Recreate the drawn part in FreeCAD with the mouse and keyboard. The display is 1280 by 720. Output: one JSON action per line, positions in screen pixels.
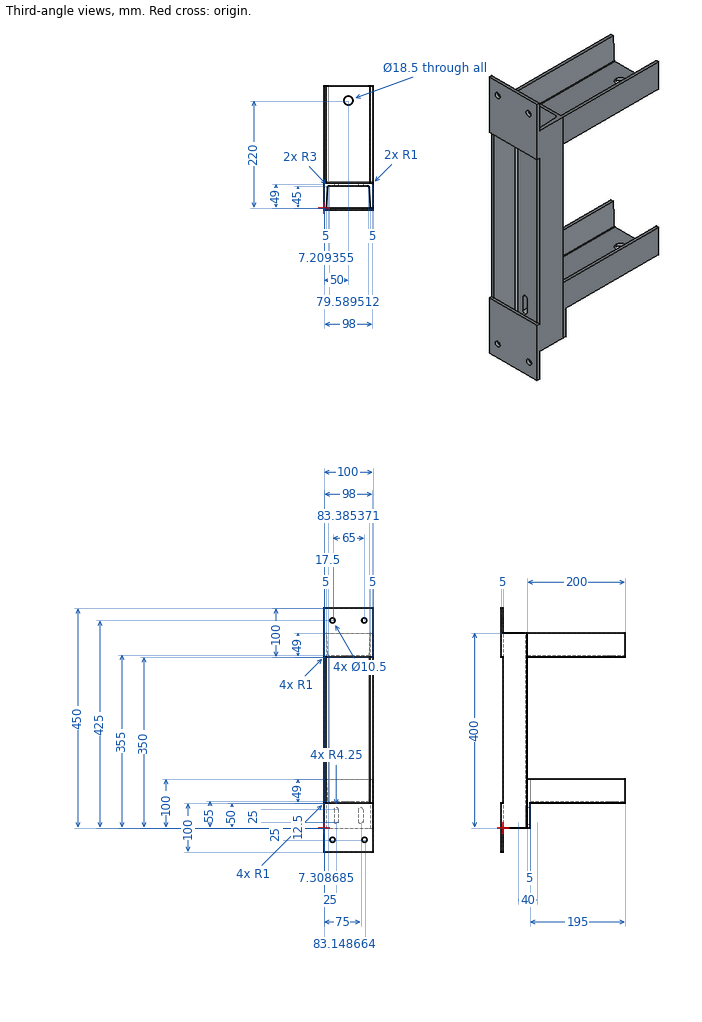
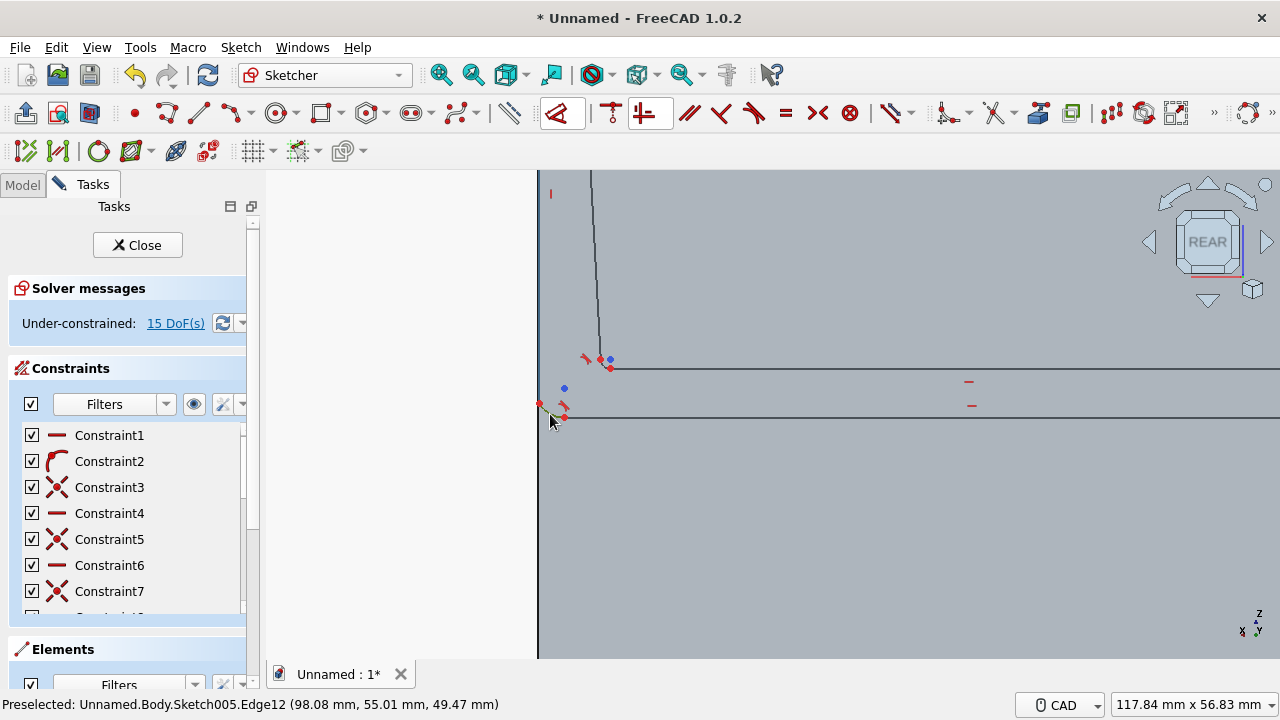
{"action": "left_click", "coordinate": [754, 114]}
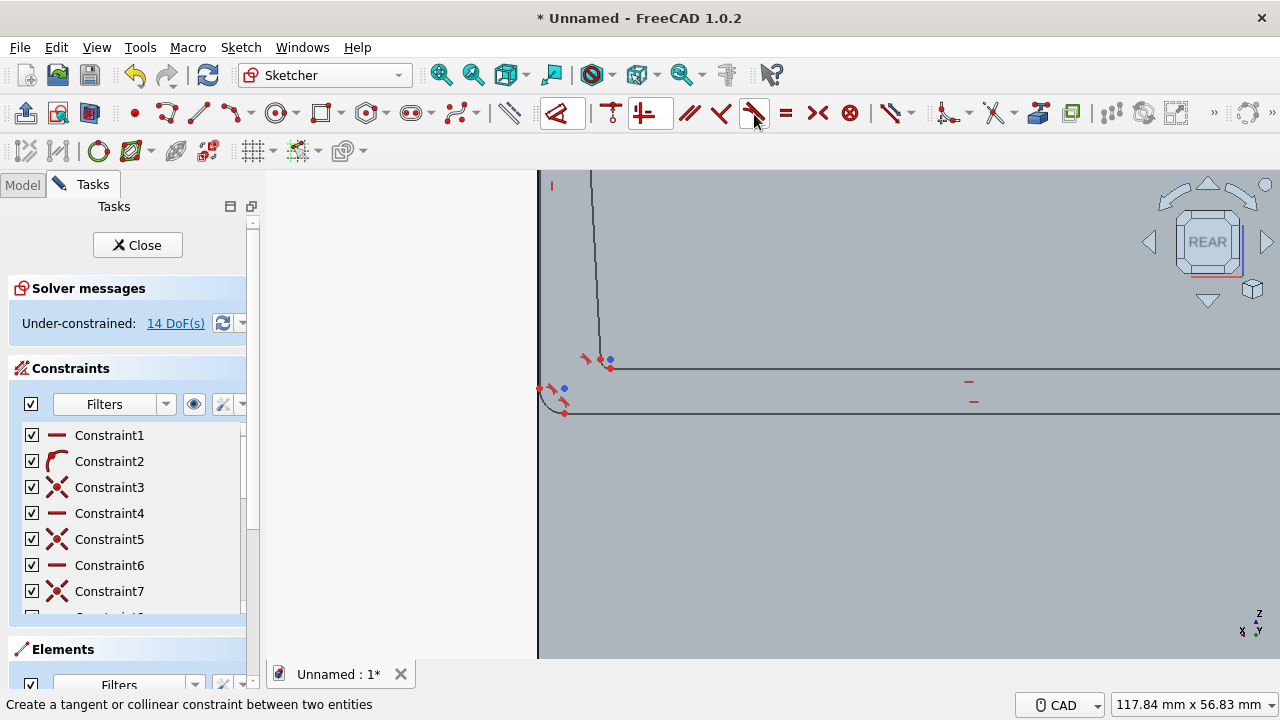
{"action": "scroll", "coordinate": [551, 416], "scroll_direction": "down", "scroll_amount": 5}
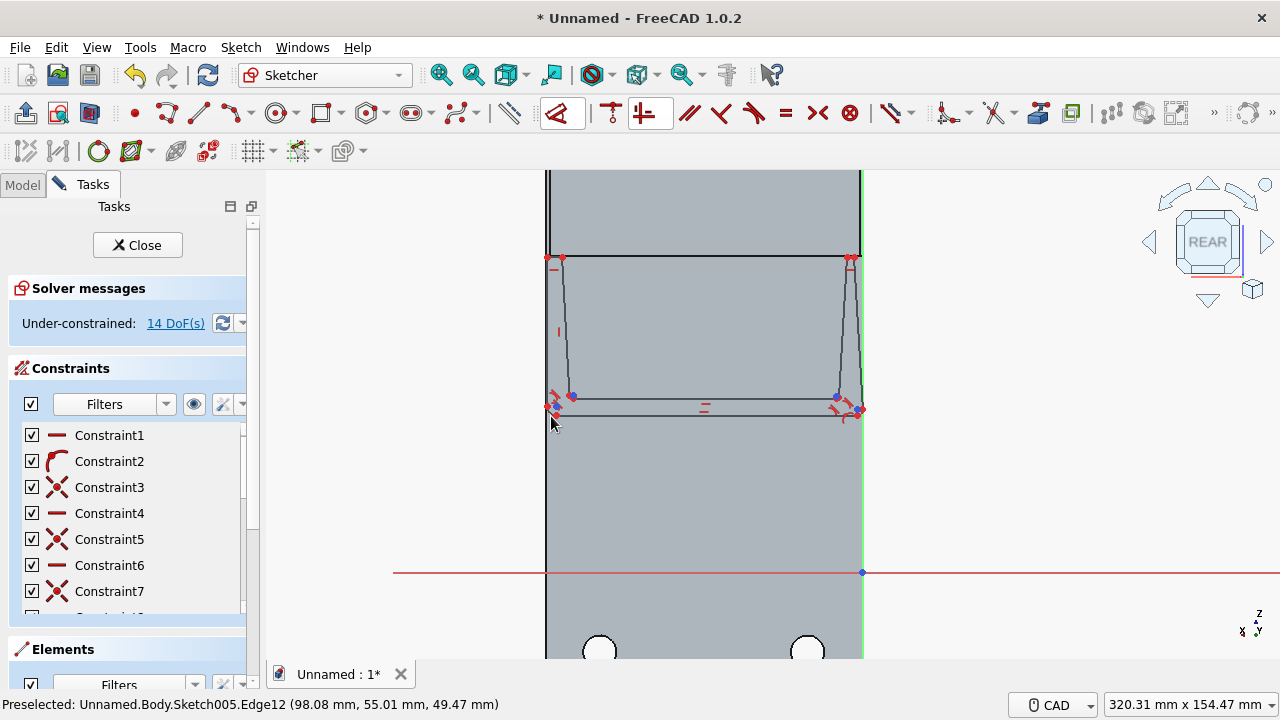
{"action": "scroll", "coordinate": [857, 303], "scroll_direction": "up", "scroll_amount": 4}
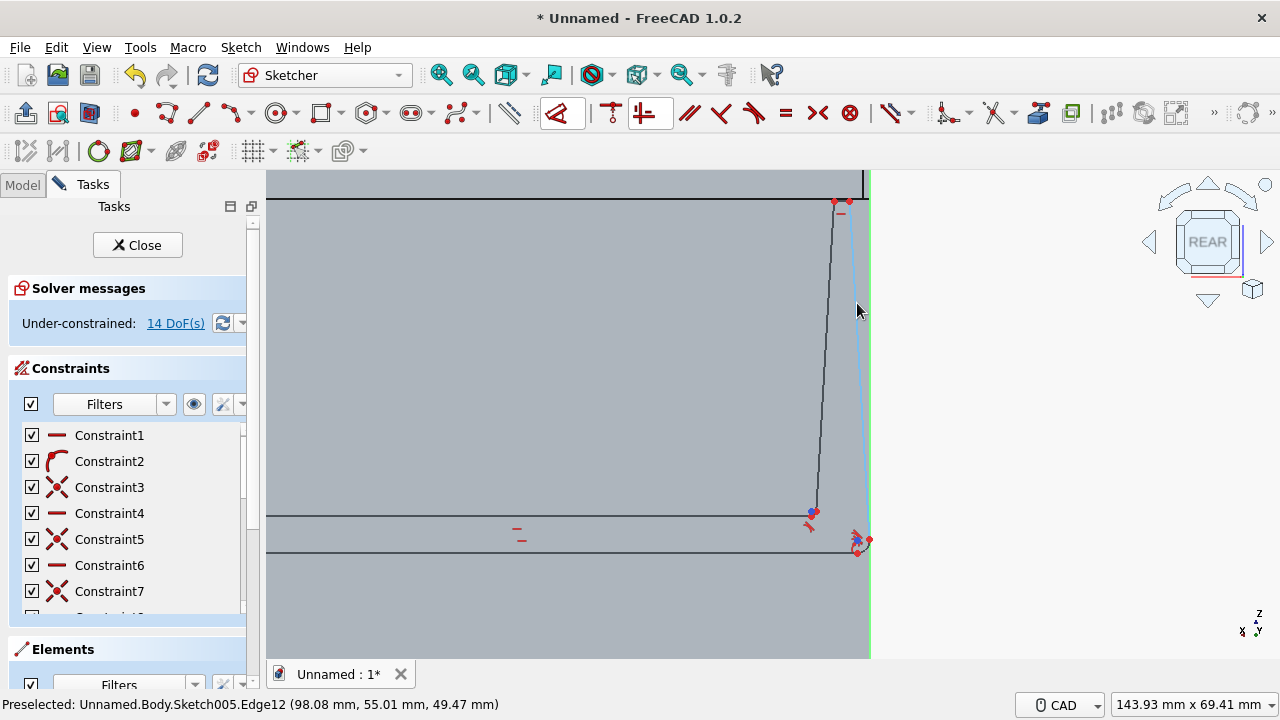
{"action": "left_click", "coordinate": [856, 303]}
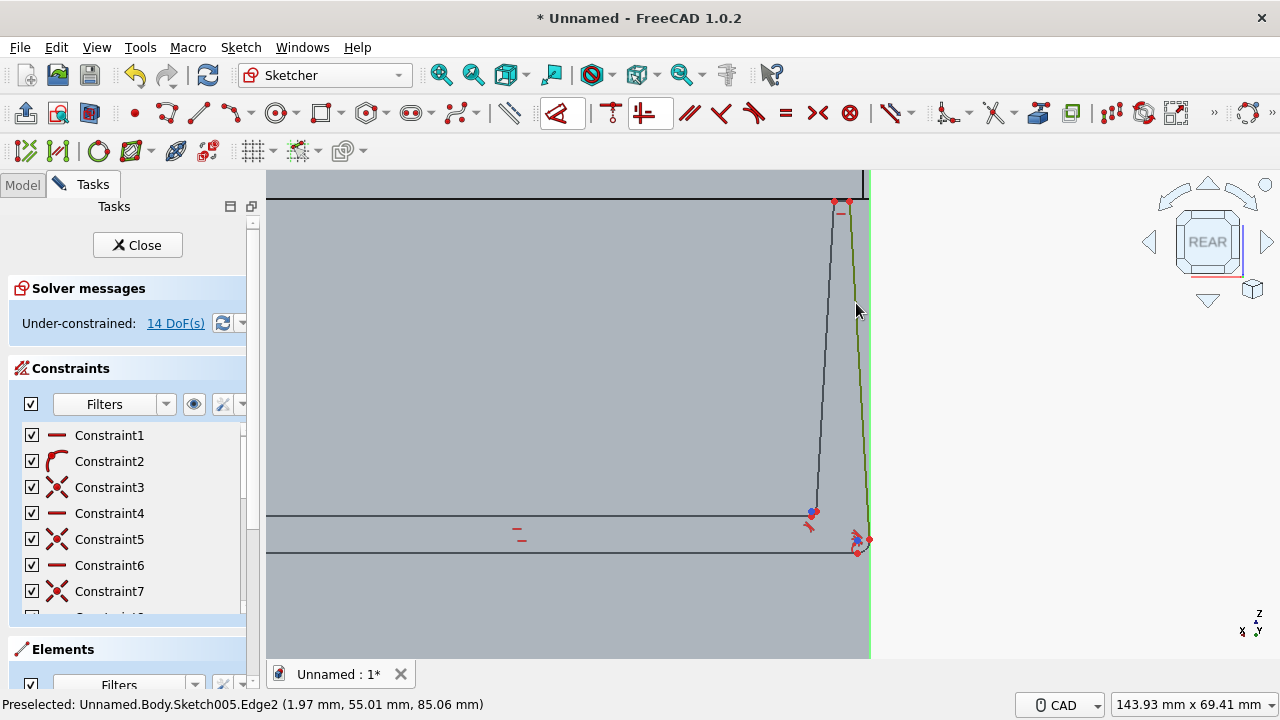
{"action": "left_click", "coordinate": [668, 114]}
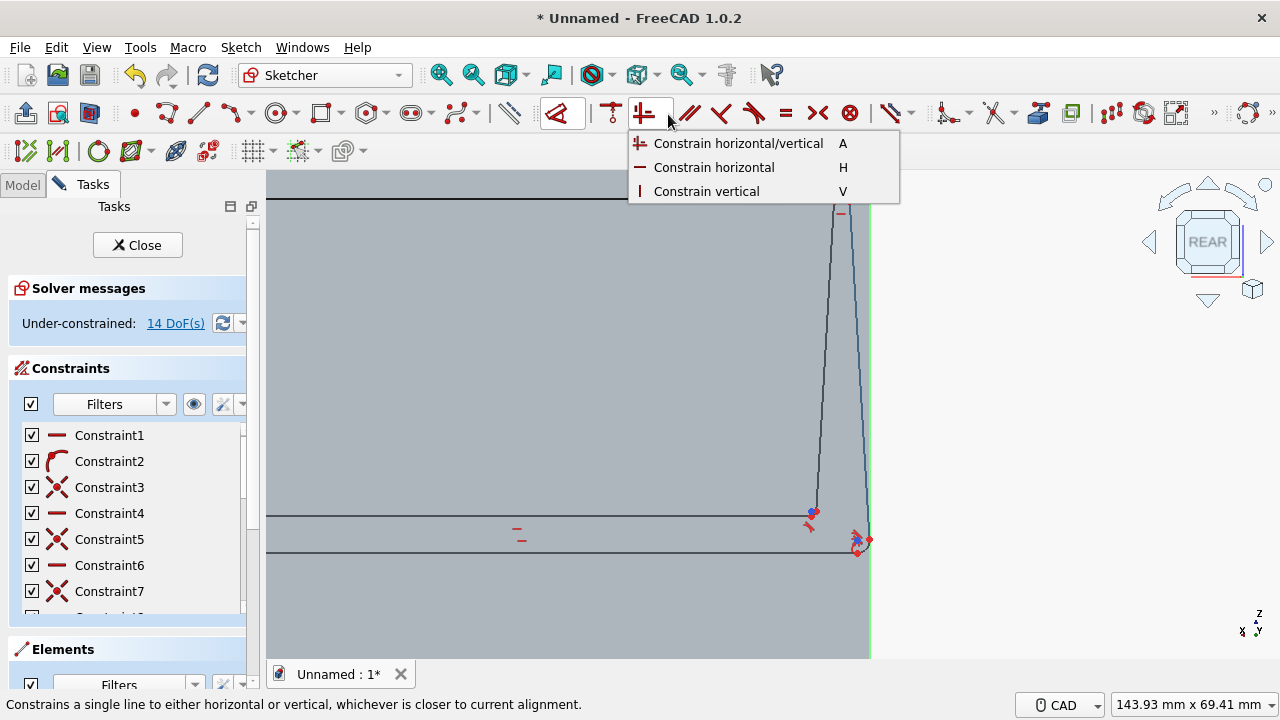
{"action": "left_click", "coordinate": [764, 191]}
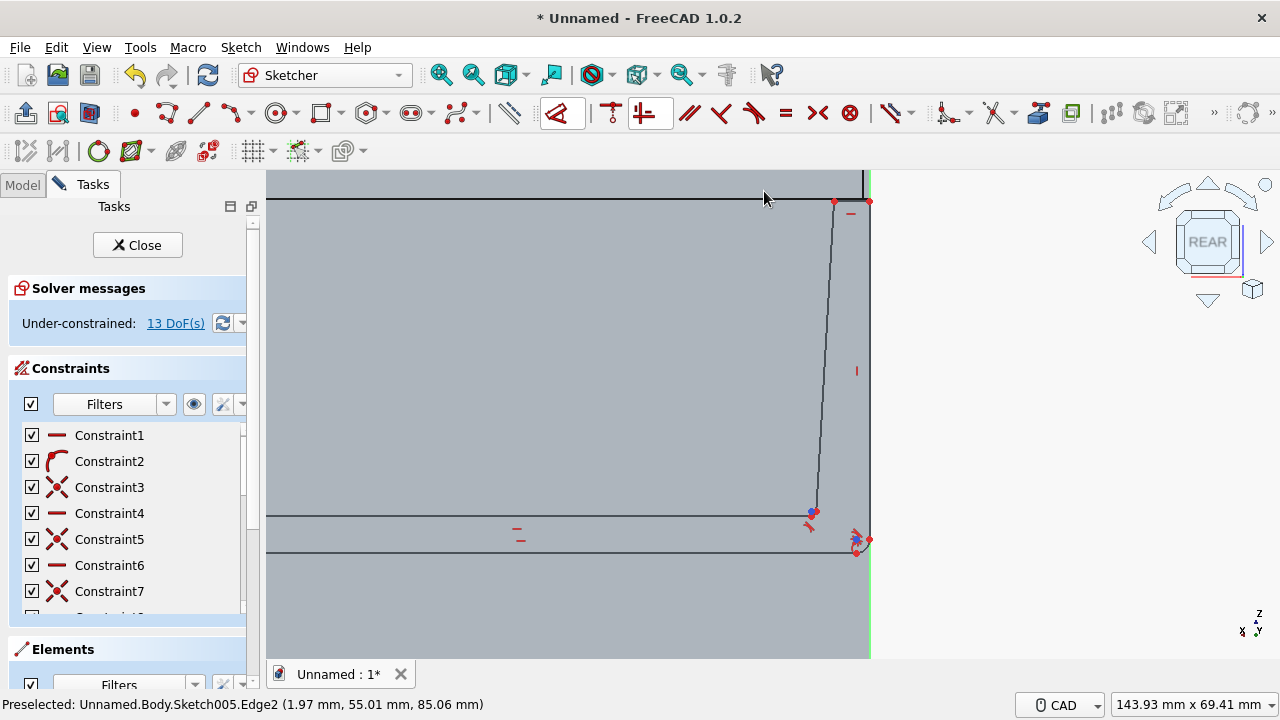
{"action": "scroll", "coordinate": [866, 549], "scroll_direction": "up", "scroll_amount": 2}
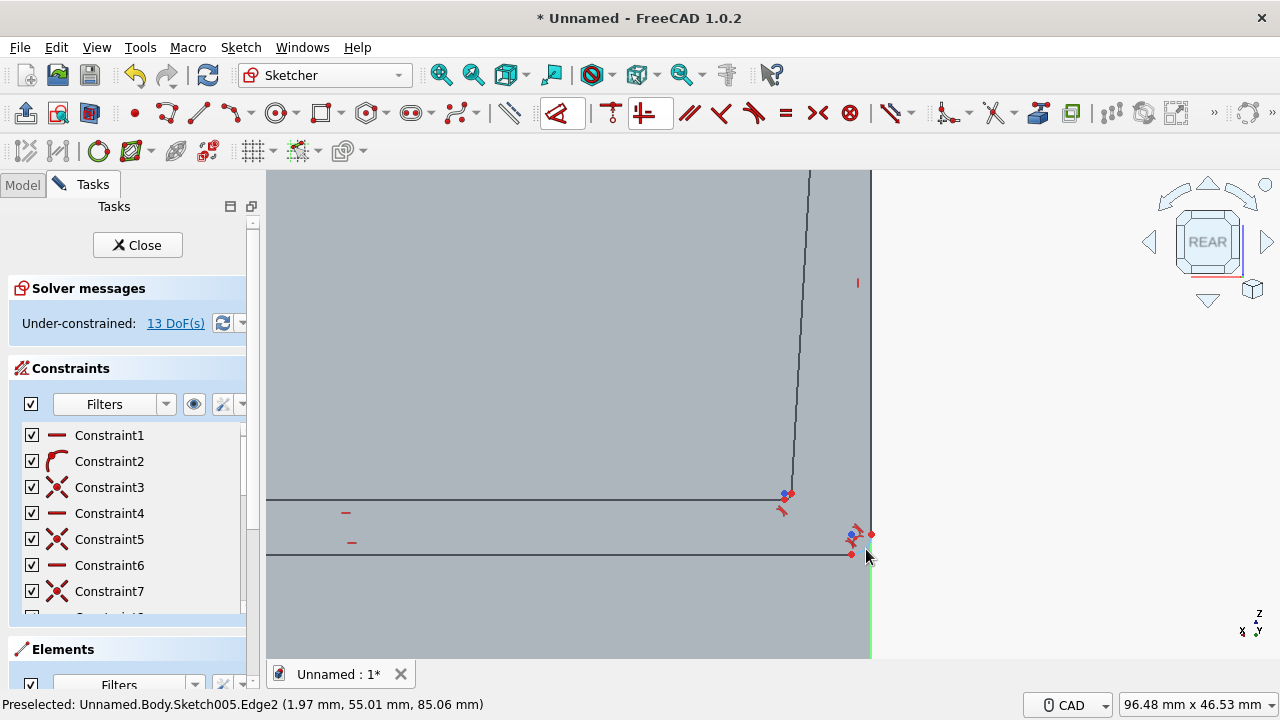
{"action": "left_click", "coordinate": [865, 549]}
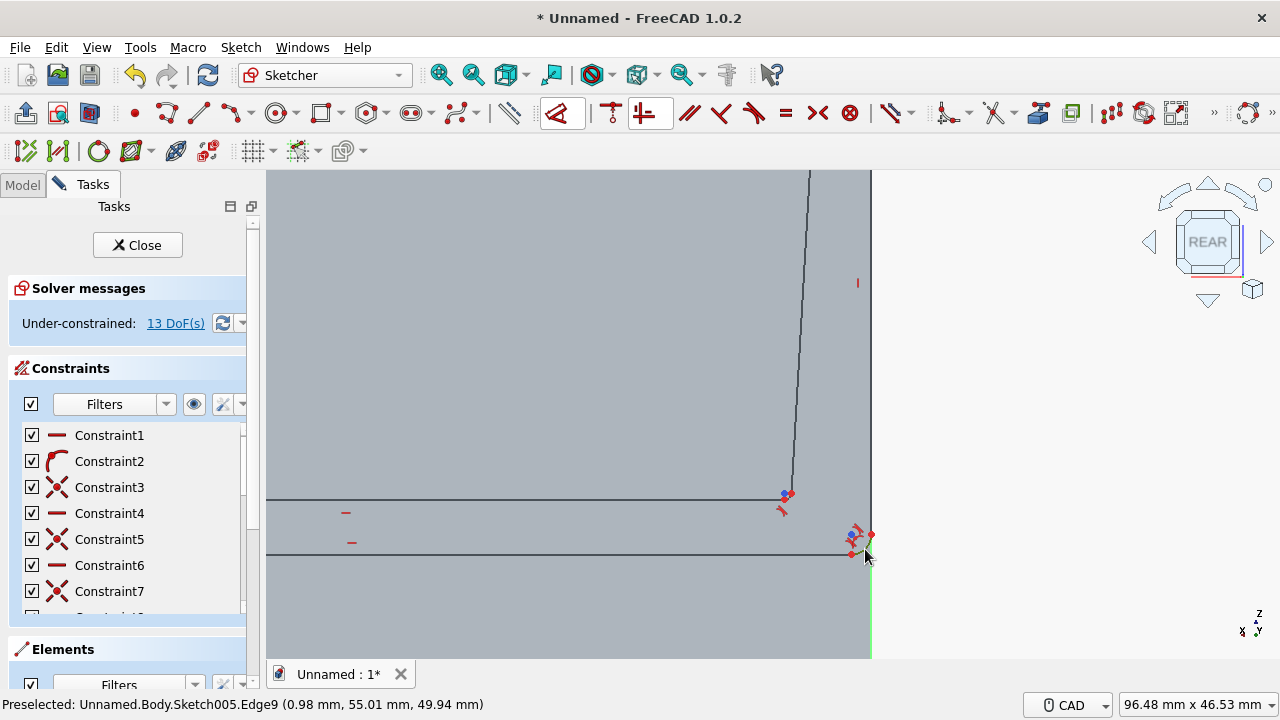
{"action": "scroll", "coordinate": [789, 498], "scroll_direction": "up", "scroll_amount": 6}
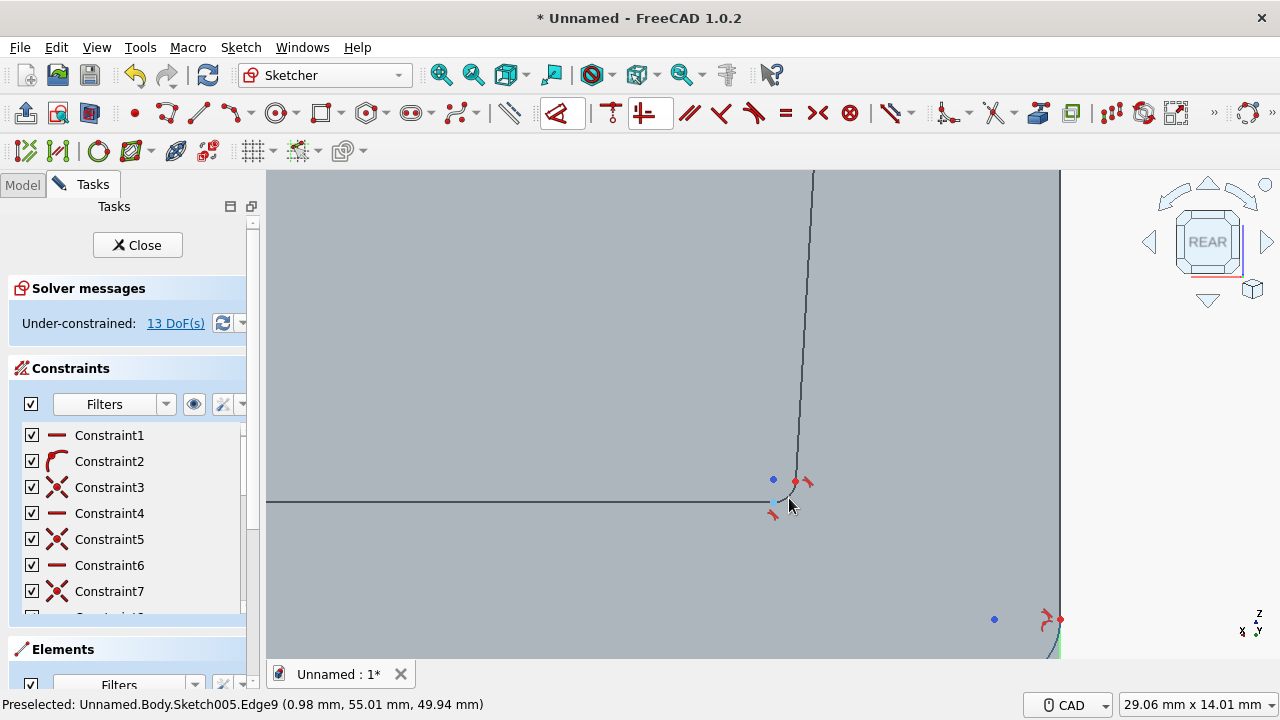
{"action": "left_click", "coordinate": [789, 496]}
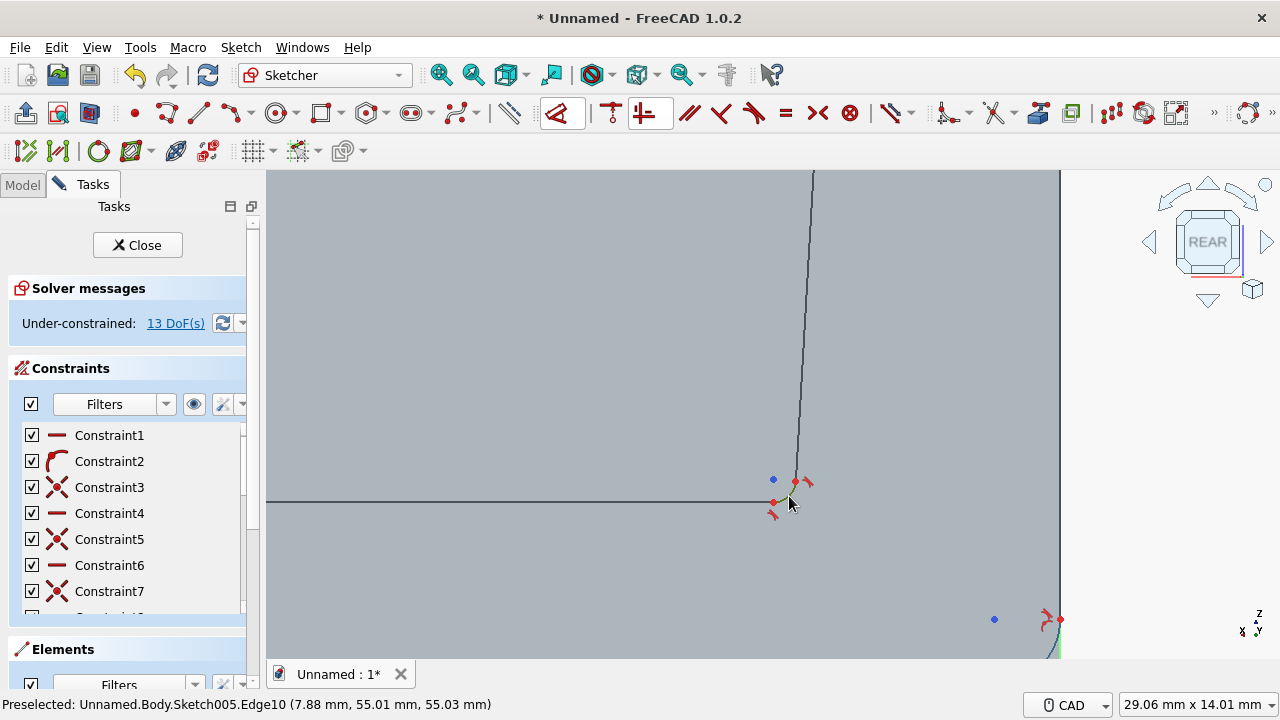
{"action": "scroll", "coordinate": [843, 389], "scroll_direction": "down", "scroll_amount": 12}